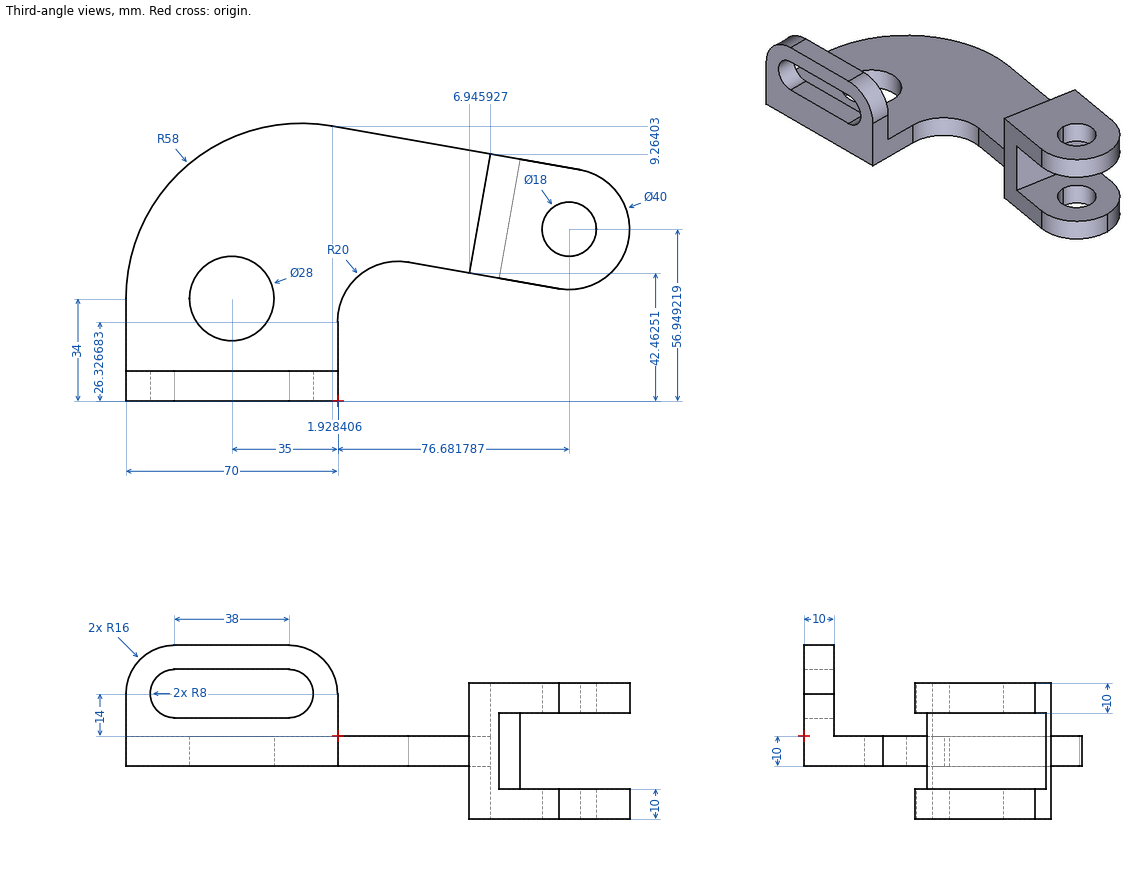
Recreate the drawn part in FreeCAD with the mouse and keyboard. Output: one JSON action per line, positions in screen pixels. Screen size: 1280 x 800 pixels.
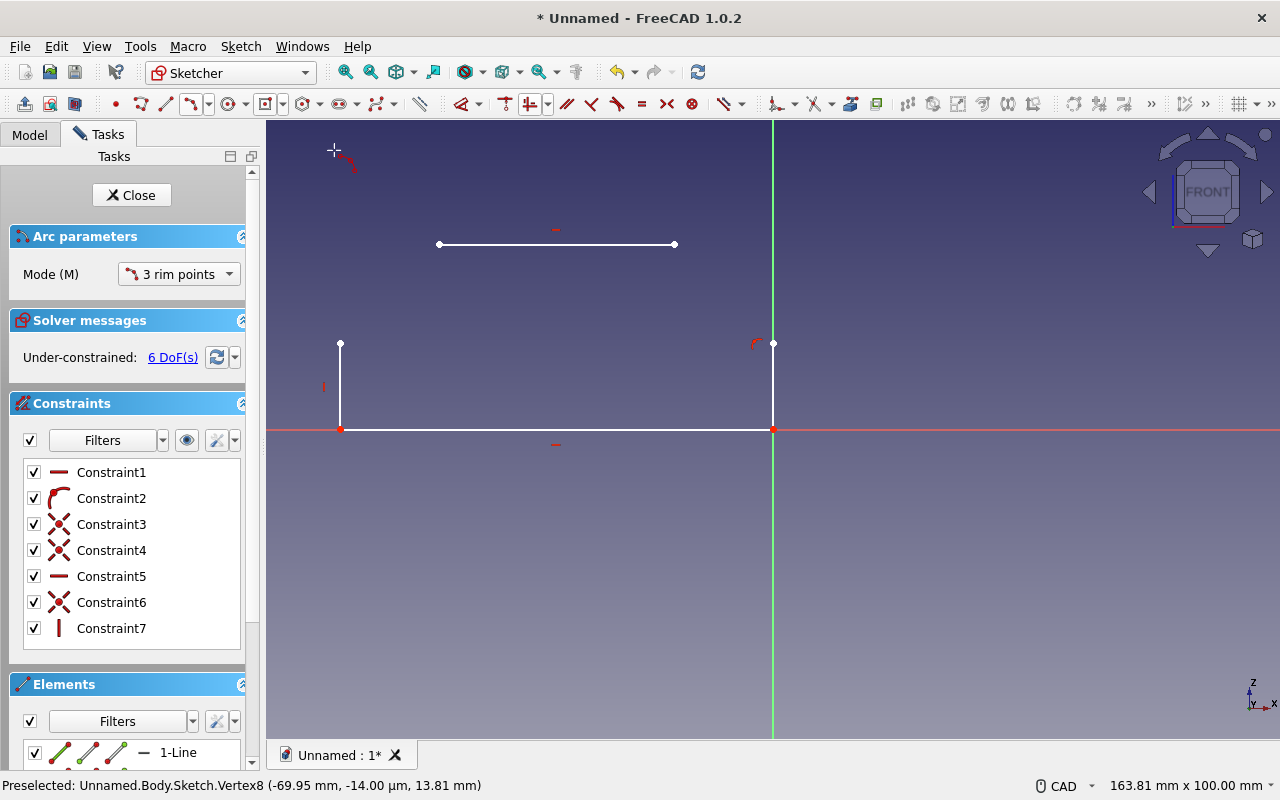
{"action": "left_click", "coordinate": [674, 245]}
{"action": "left_click", "coordinate": [773, 344]}
{"action": "left_click", "coordinate": [744, 273]}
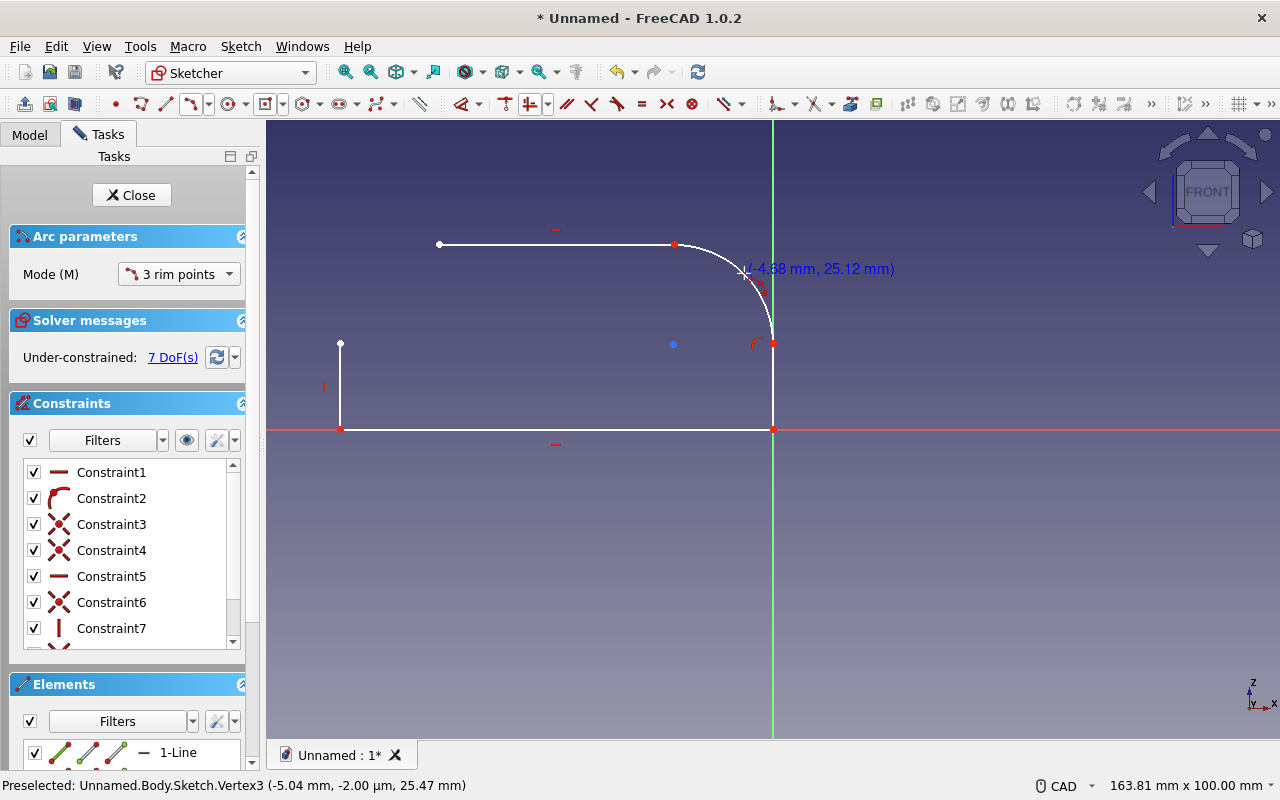
{"action": "left_click", "coordinate": [340, 344]}
{"action": "left_click", "coordinate": [439, 245]}
{"action": "left_click", "coordinate": [369, 273]}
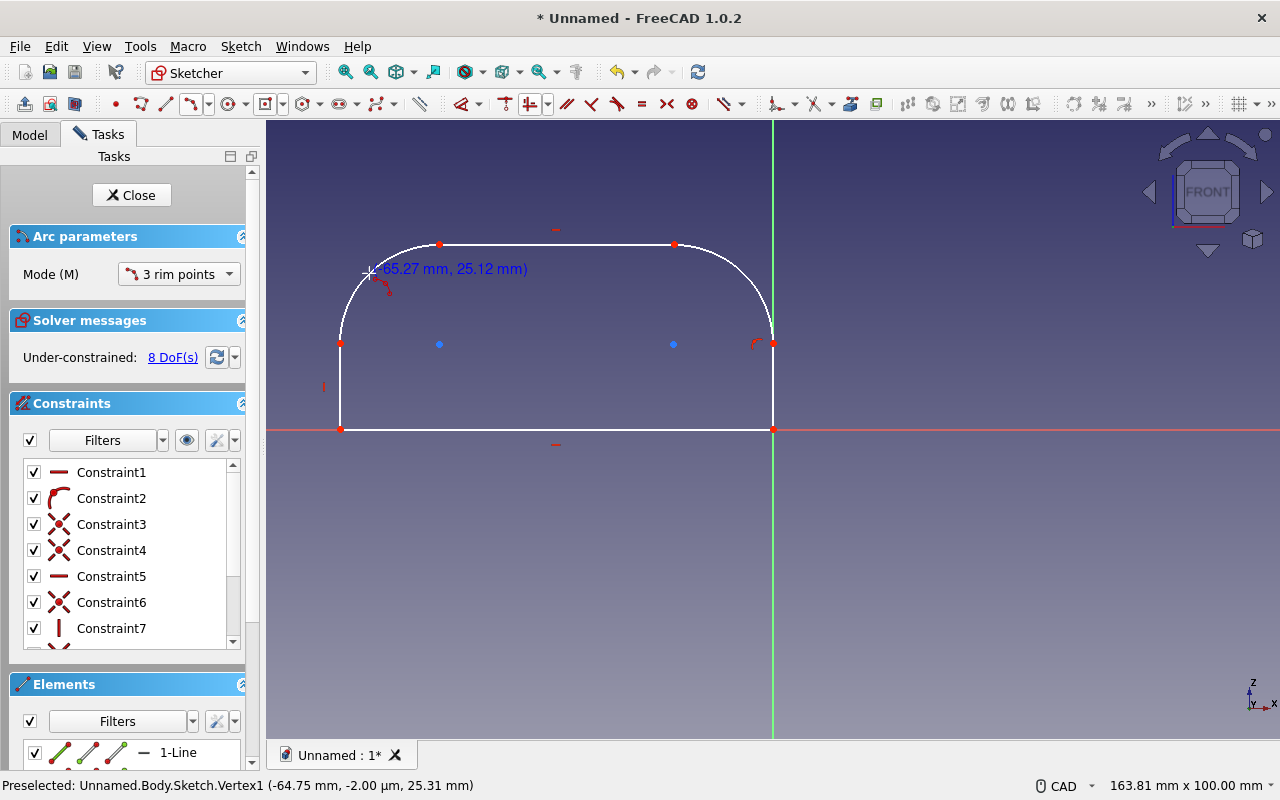
{"action": "left_click", "coordinate": [338, 104]}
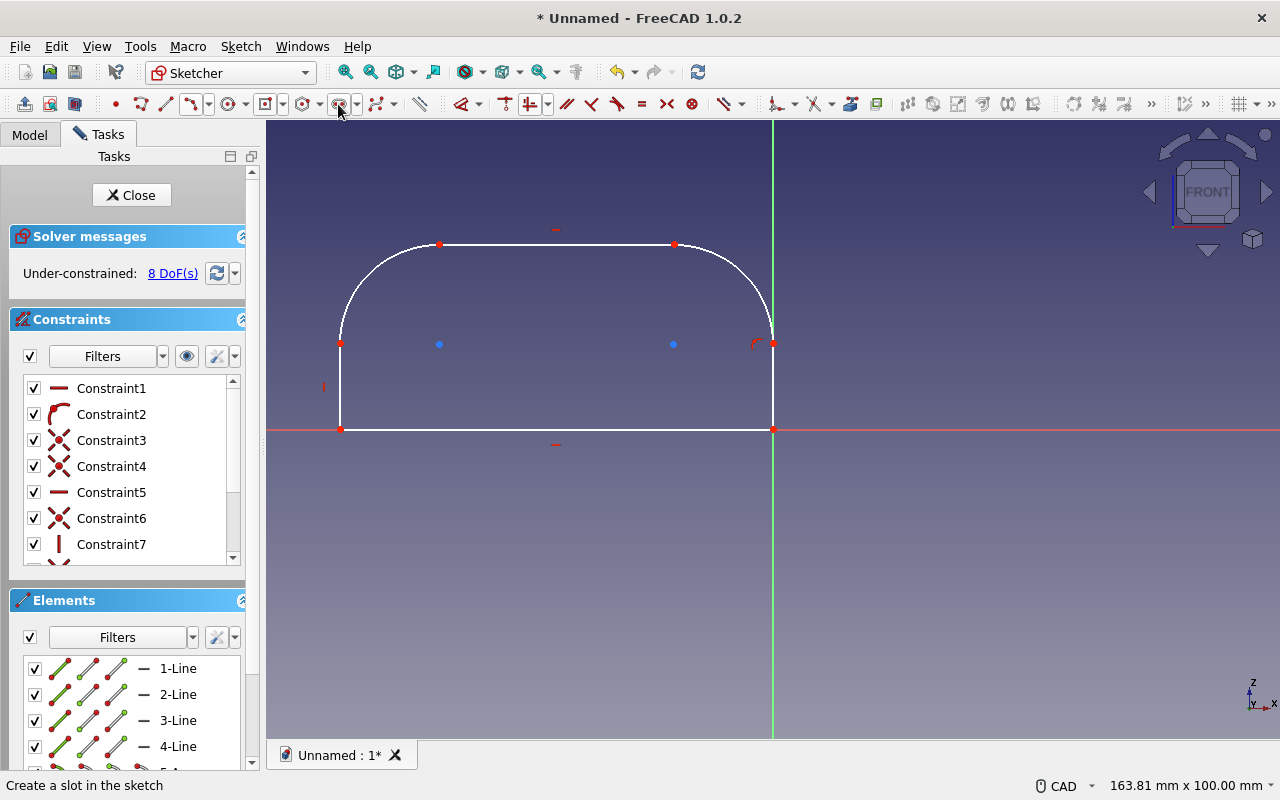
{"action": "left_click", "coordinate": [439, 343]}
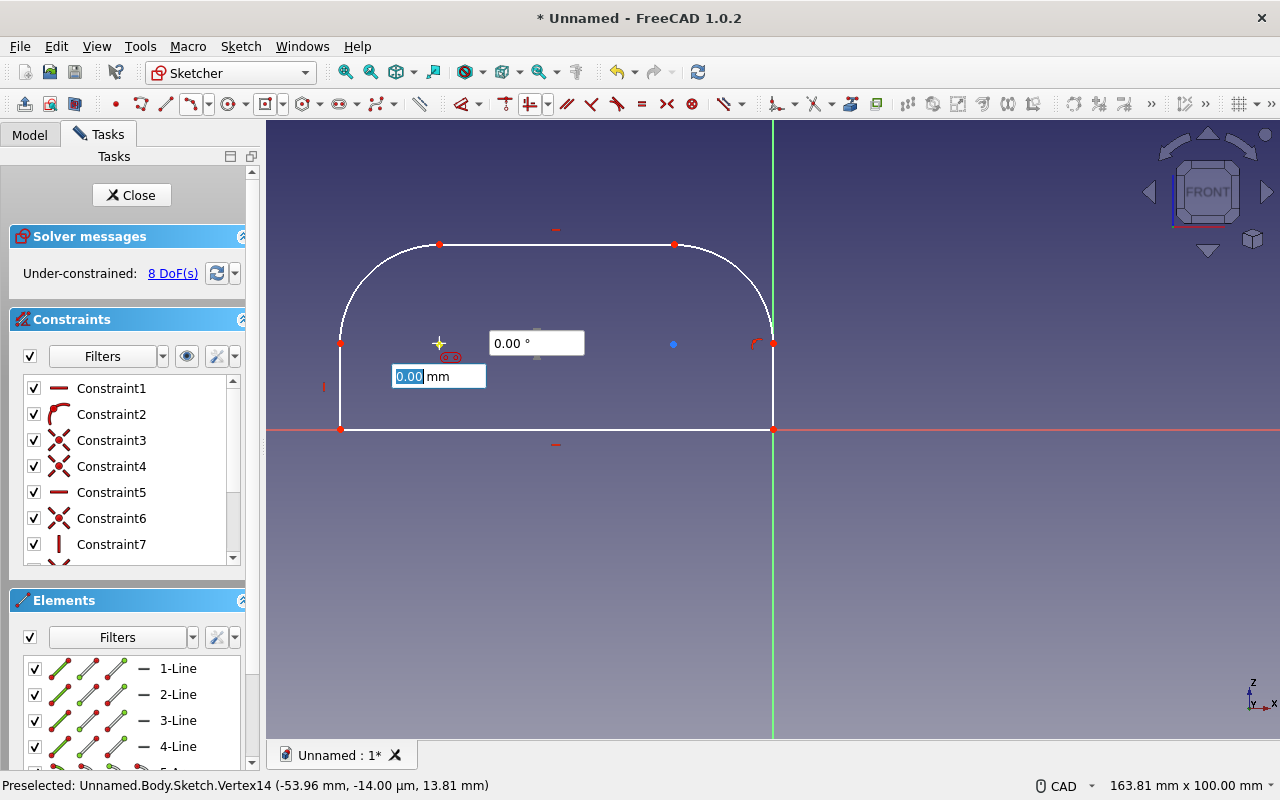
{"action": "left_click", "coordinate": [674, 343]}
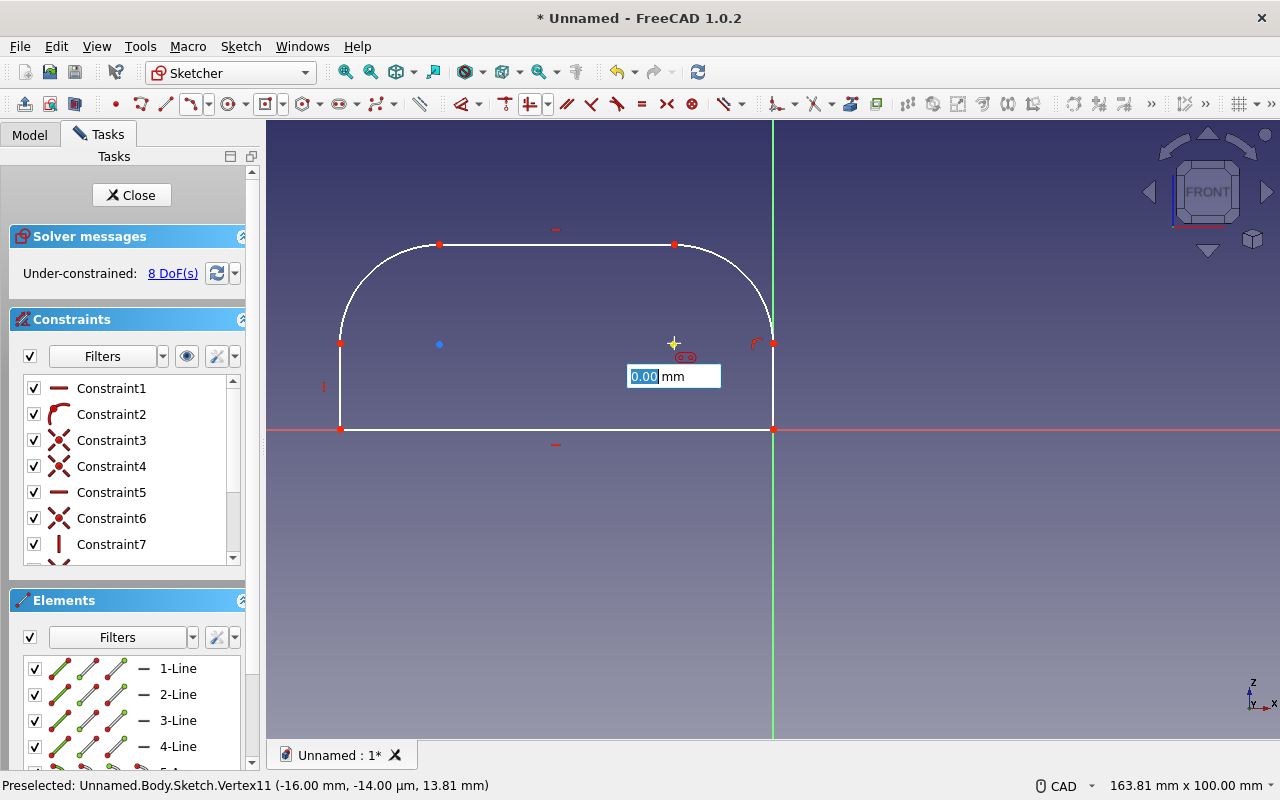
{"action": "left_click", "coordinate": [556, 392]}
{"action": "key", "text": "Escape"}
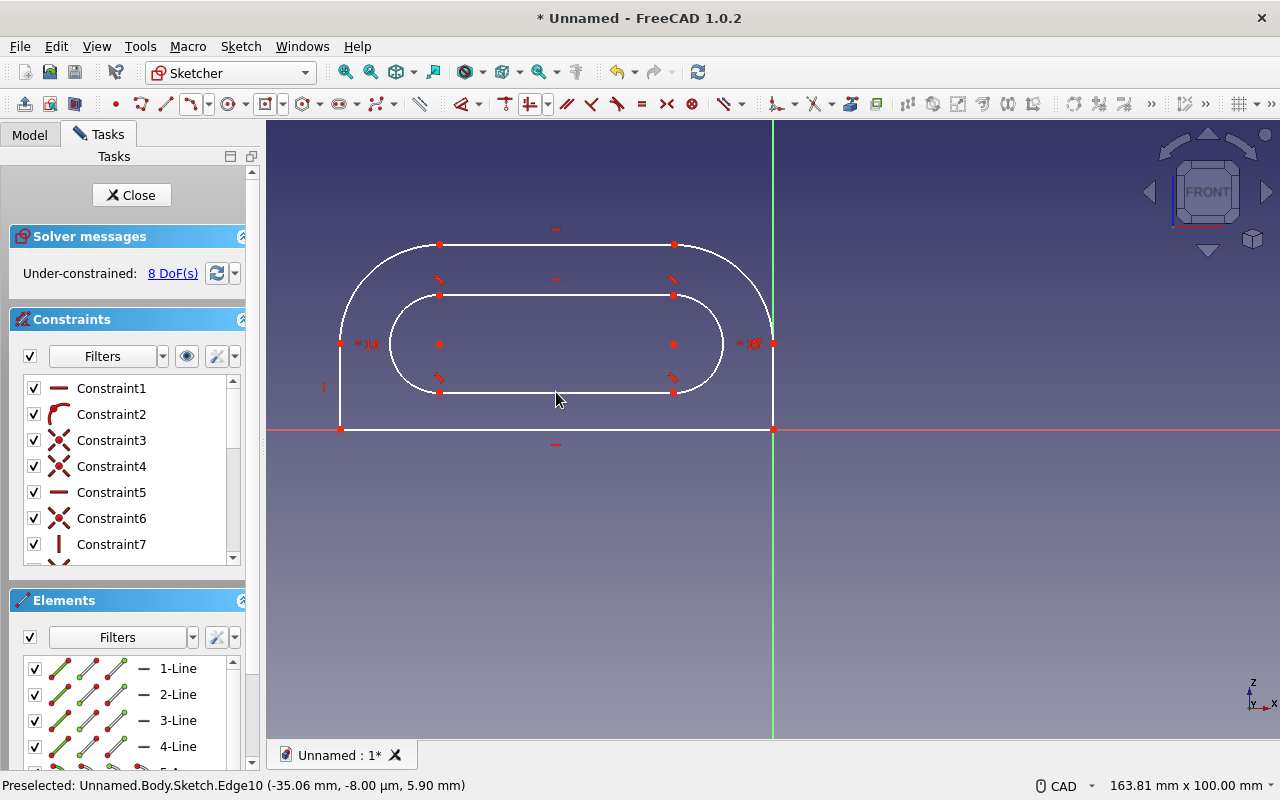
{"action": "left_click", "coordinate": [509, 245]}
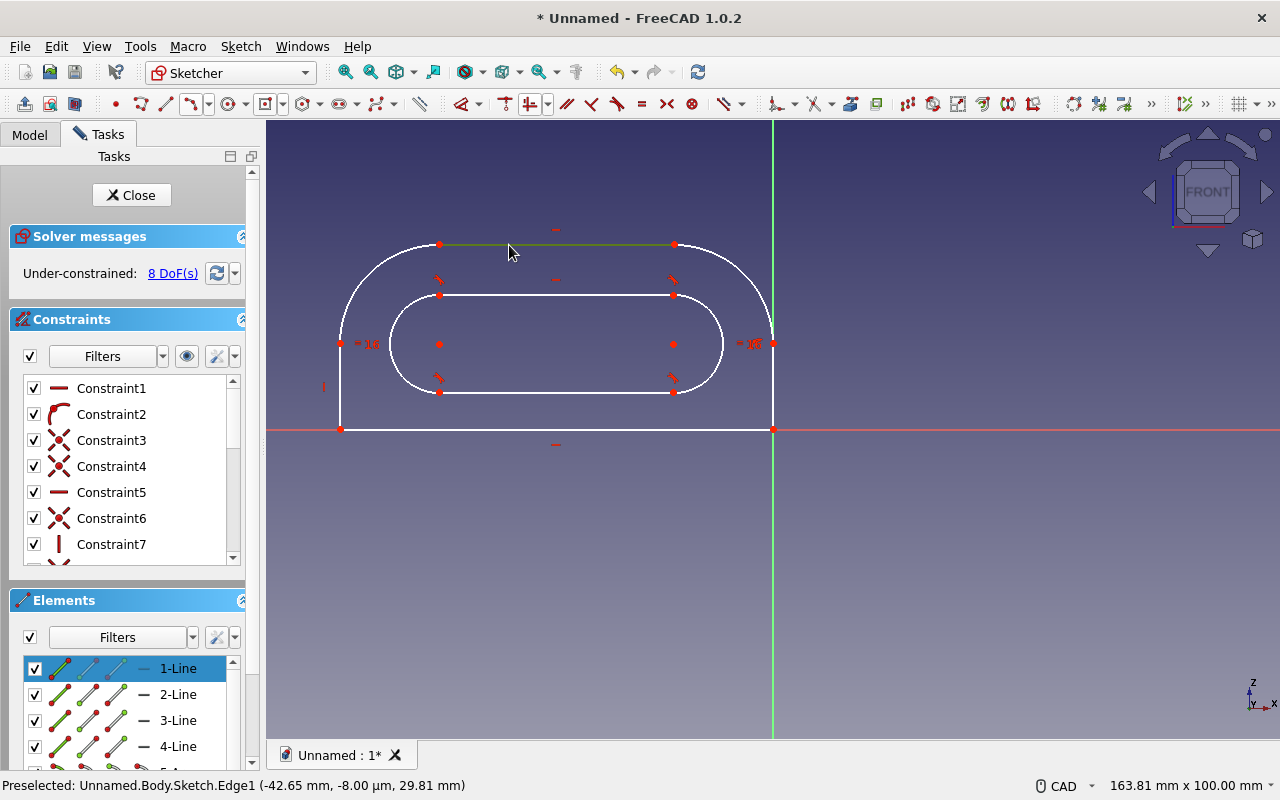
{"action": "scroll", "coordinate": [762, 299], "scroll_direction": "up", "scroll_amount": 2}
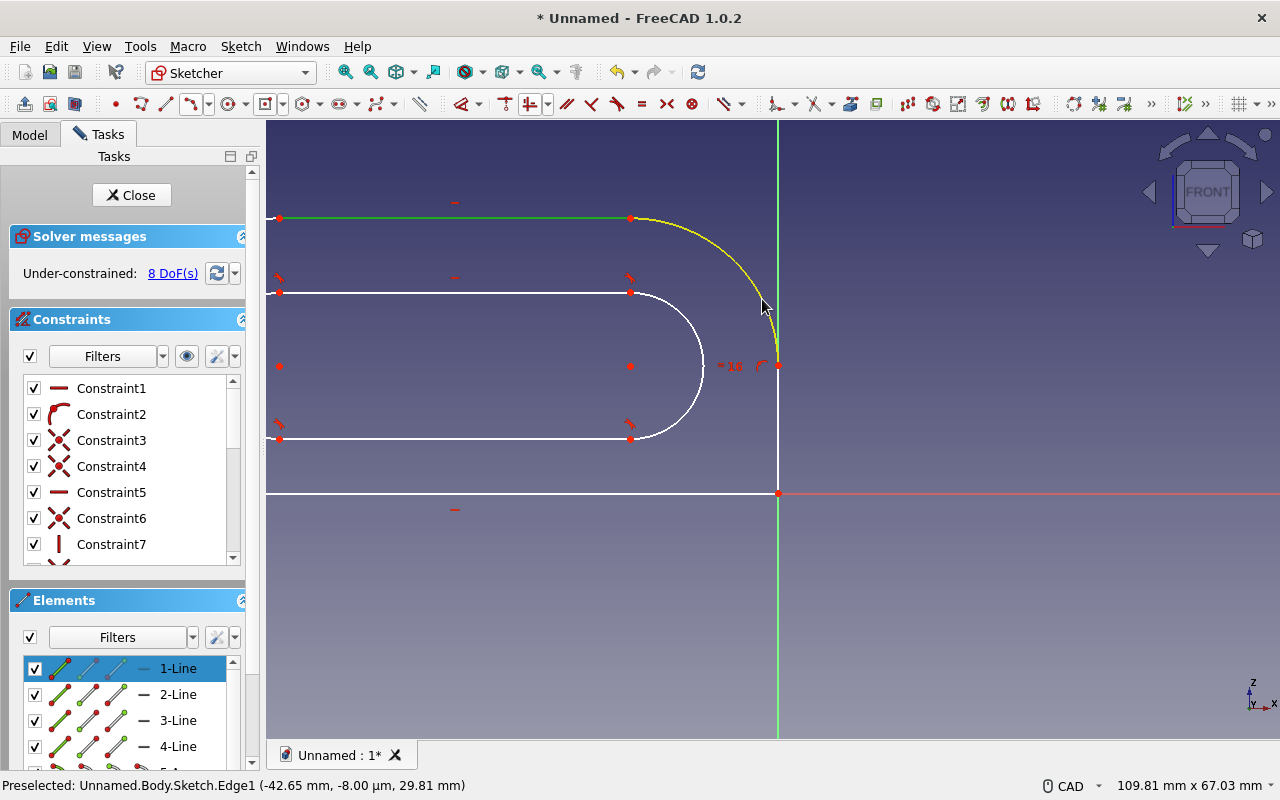
{"action": "left_click", "coordinate": [762, 299]}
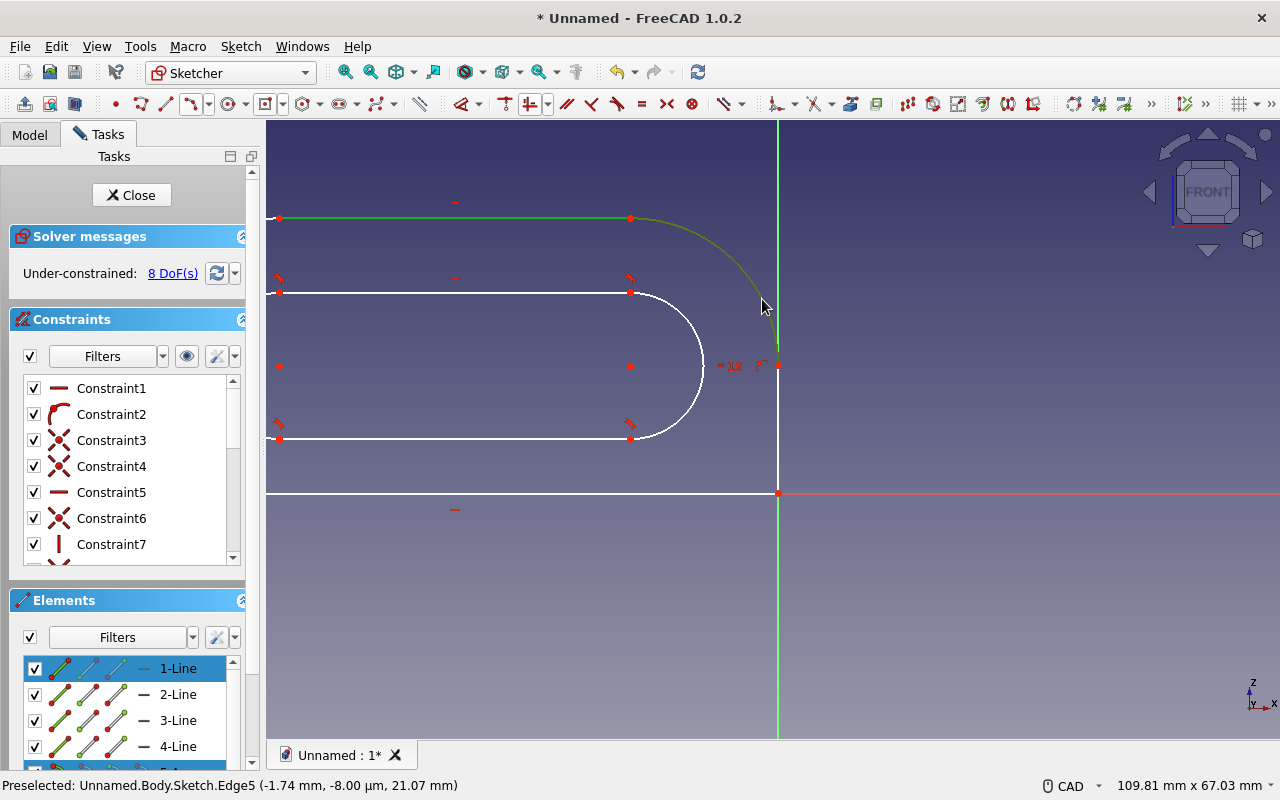
{"action": "left_click", "coordinate": [617, 104]}